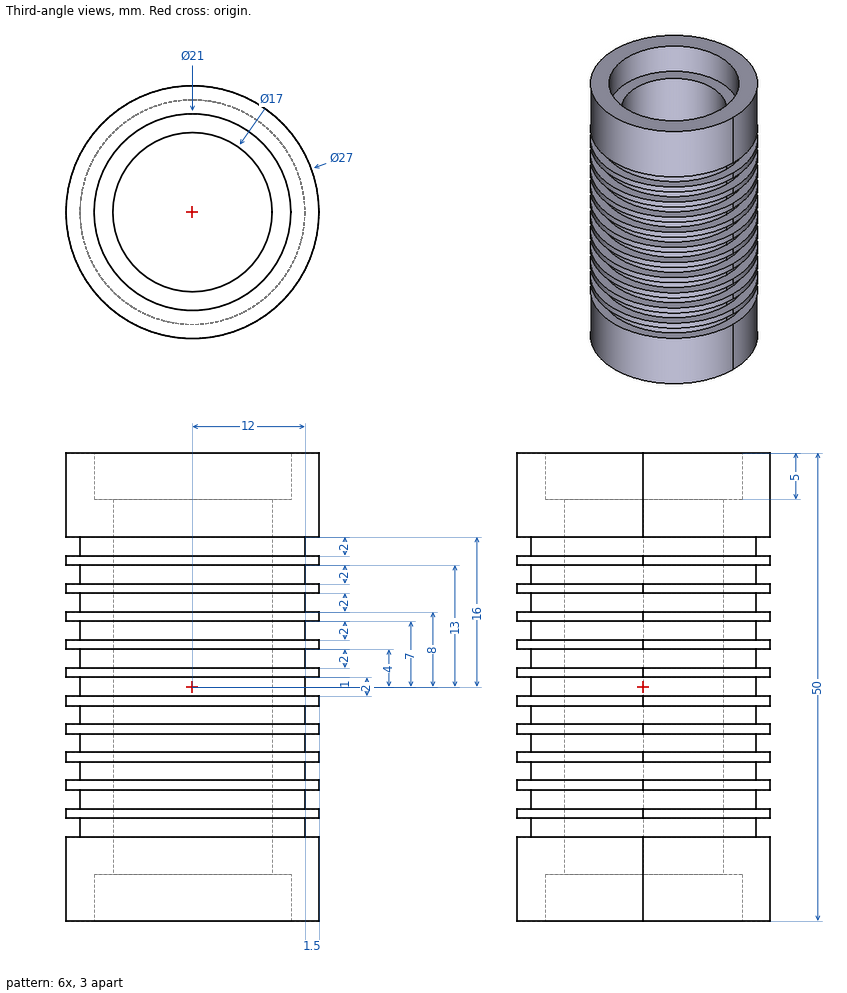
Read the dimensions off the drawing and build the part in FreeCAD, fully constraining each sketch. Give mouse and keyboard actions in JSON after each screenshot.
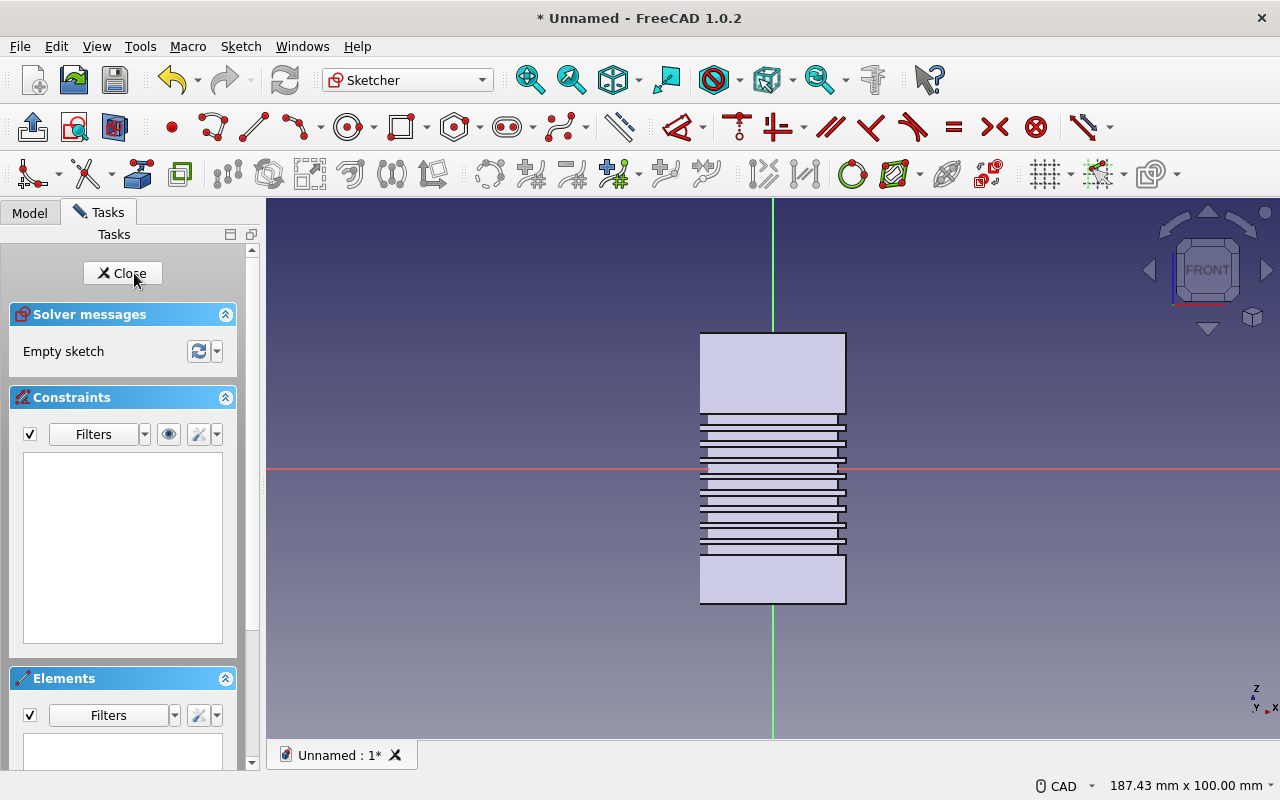
{"action": "left_click", "coordinate": [115, 128]}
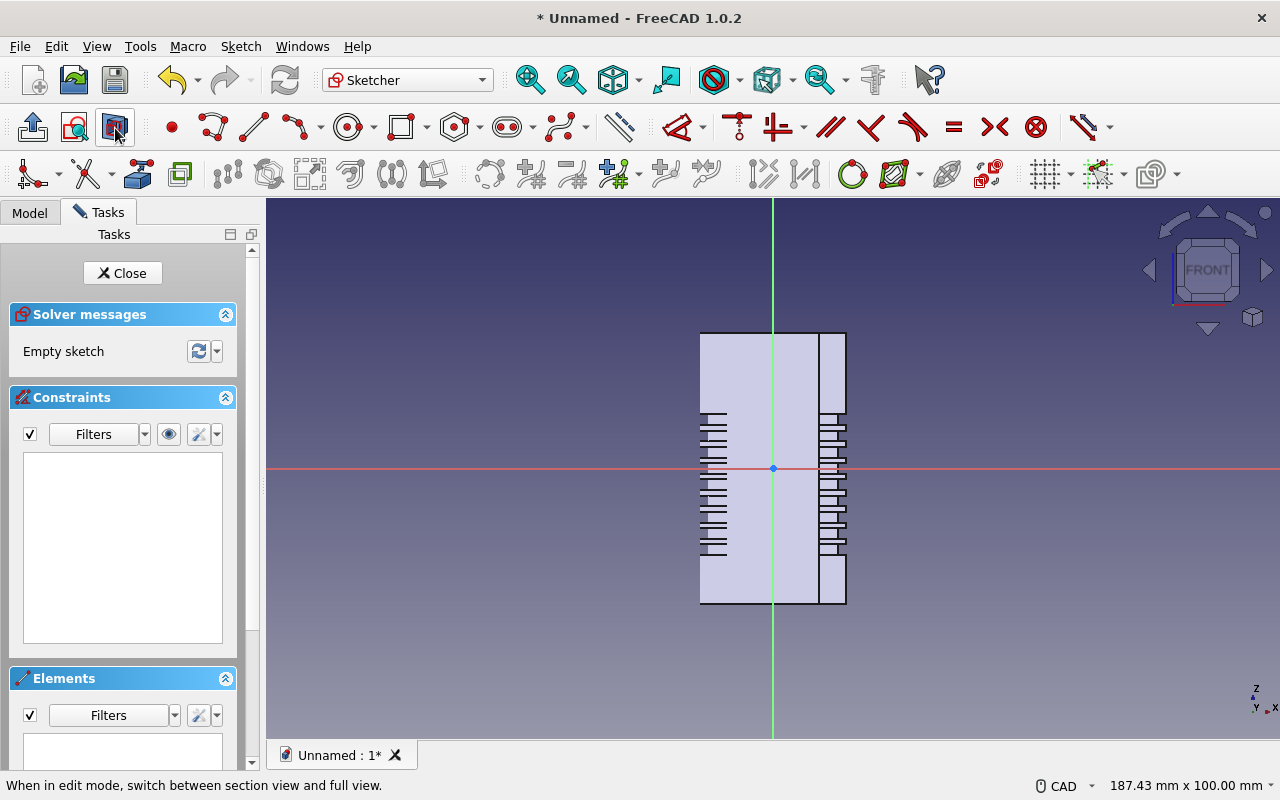
{"action": "scroll", "coordinate": [849, 400], "scroll_direction": "up", "scroll_amount": 15}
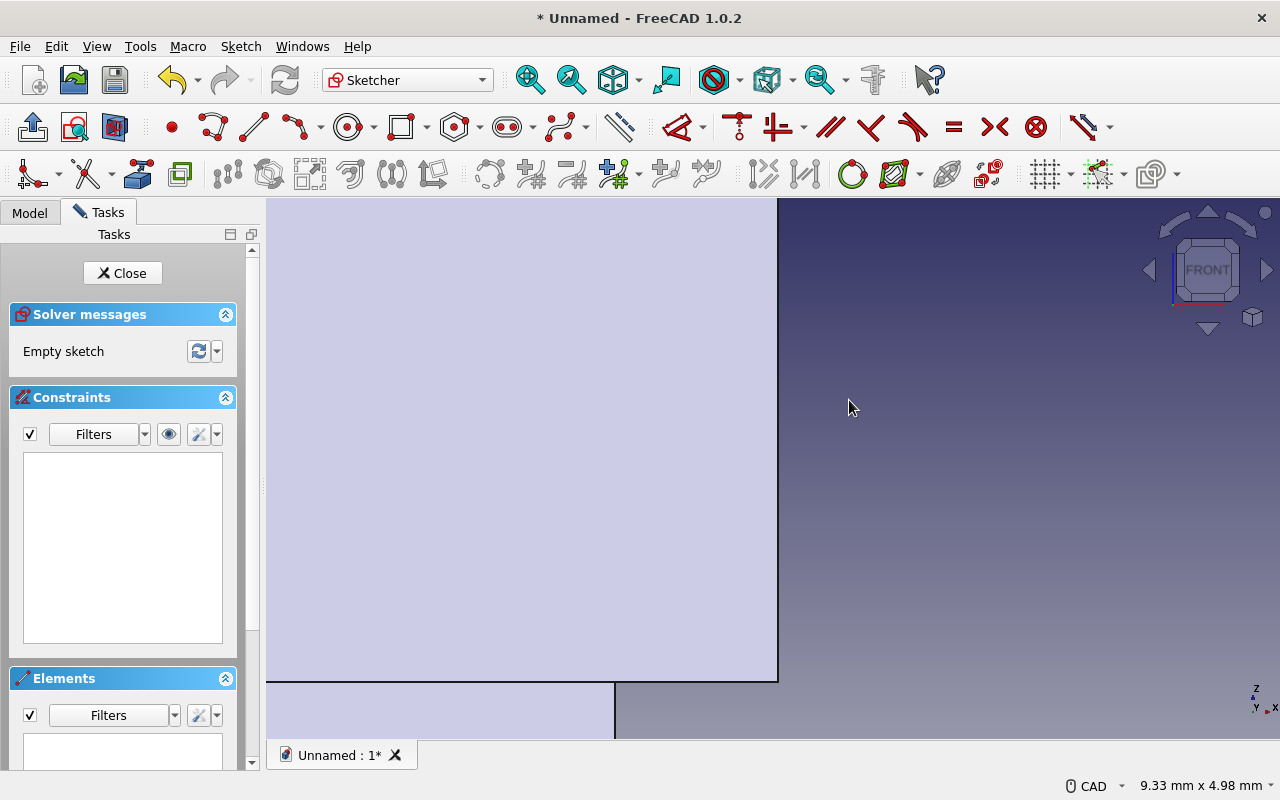
{"action": "scroll", "coordinate": [682, 457], "scroll_direction": "up", "scroll_amount": 2}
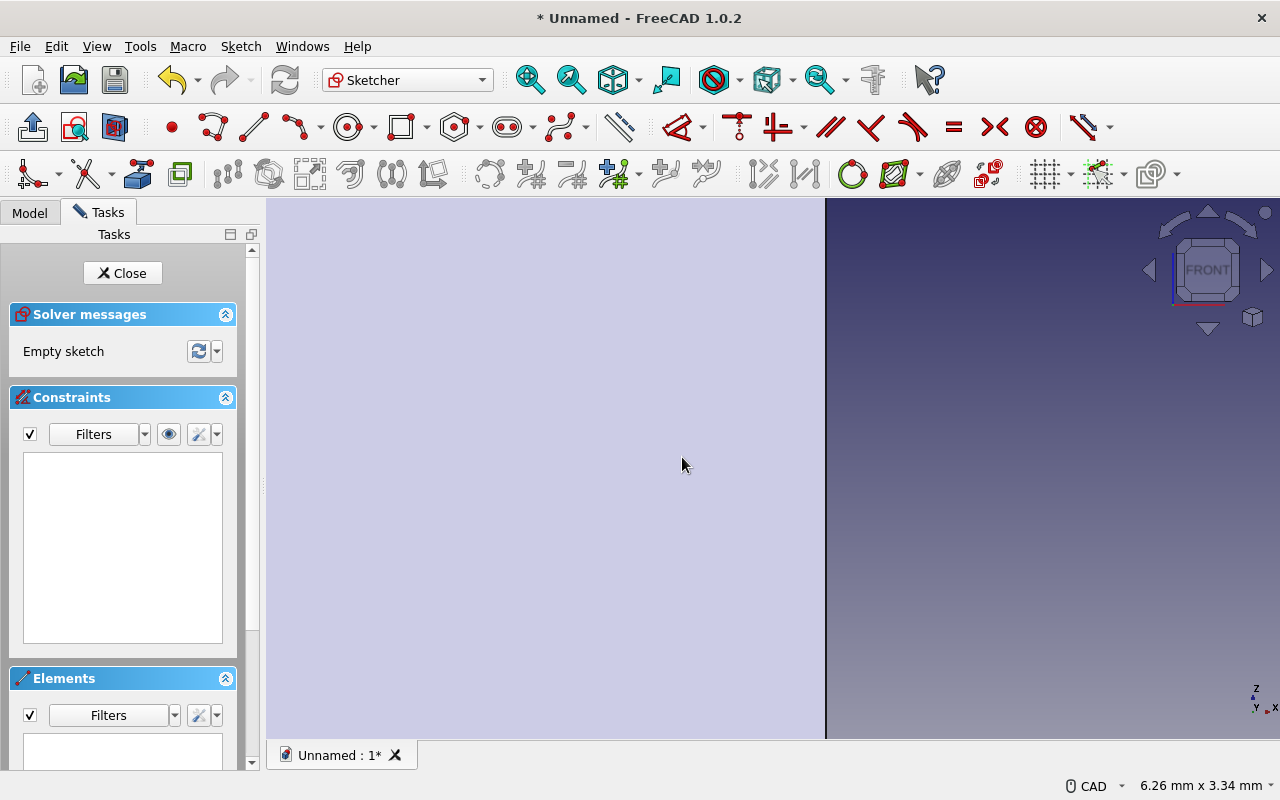
{"action": "key", "text": "g r"}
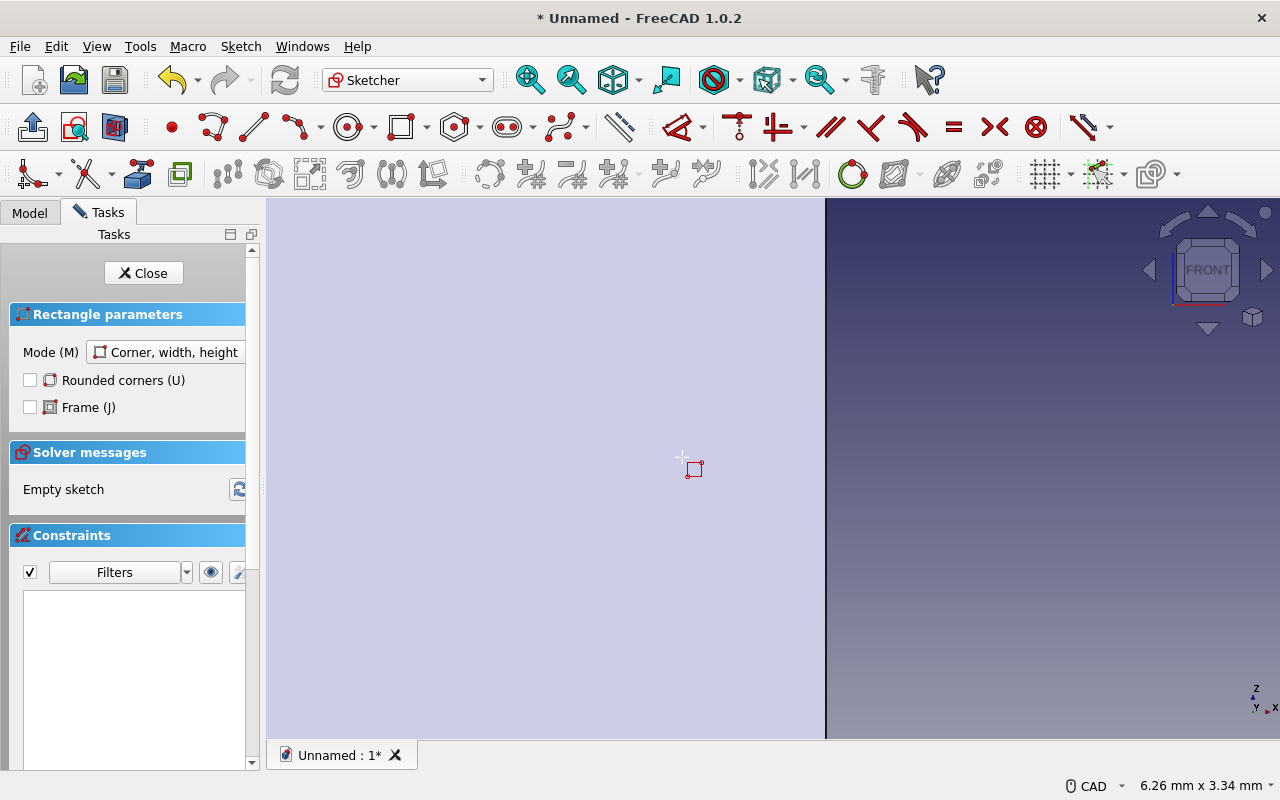
{"action": "left_click", "coordinate": [583, 306]}
{"action": "mouse_move", "coordinate": [826, 630]}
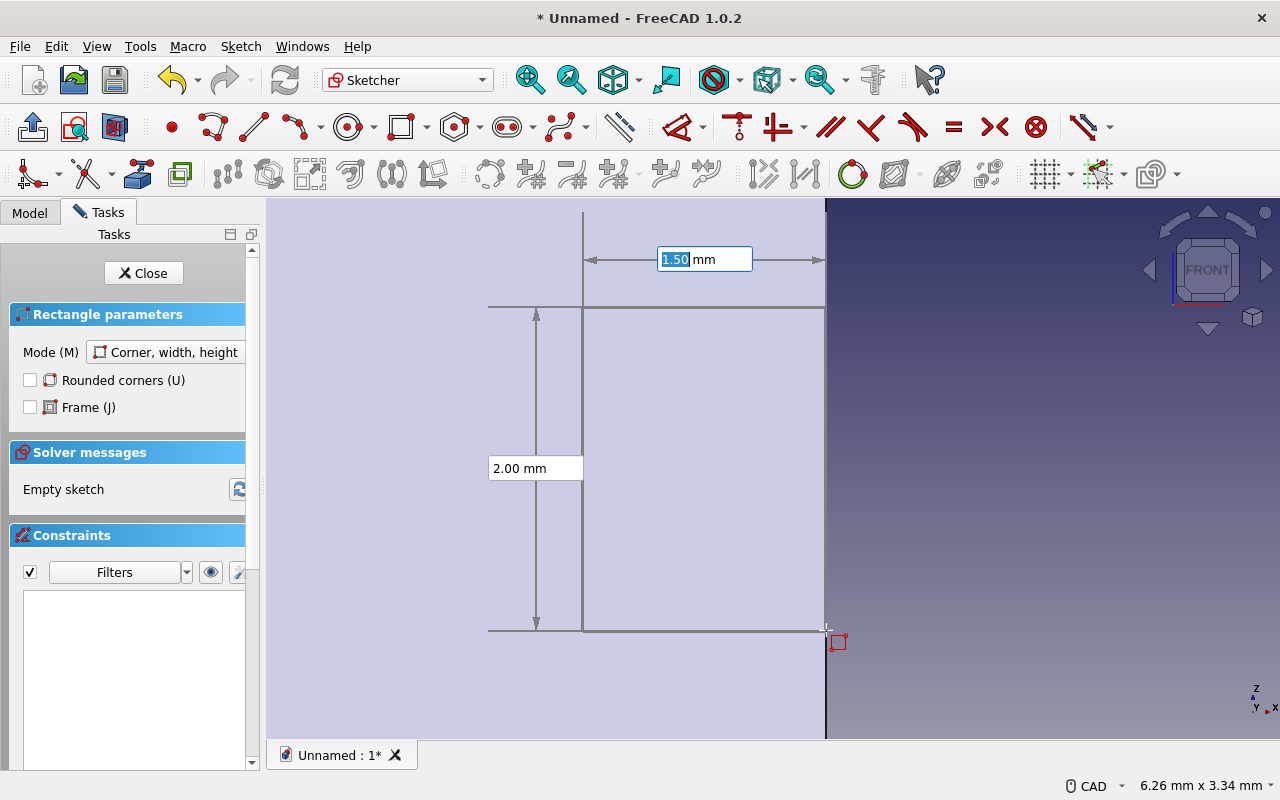
{"action": "type", "text": "1.5"}
{"action": "key", "text": "Tab"}
{"action": "type", "text": "2"}
{"action": "key", "text": "Return"}
{"action": "key", "text": "Escape"}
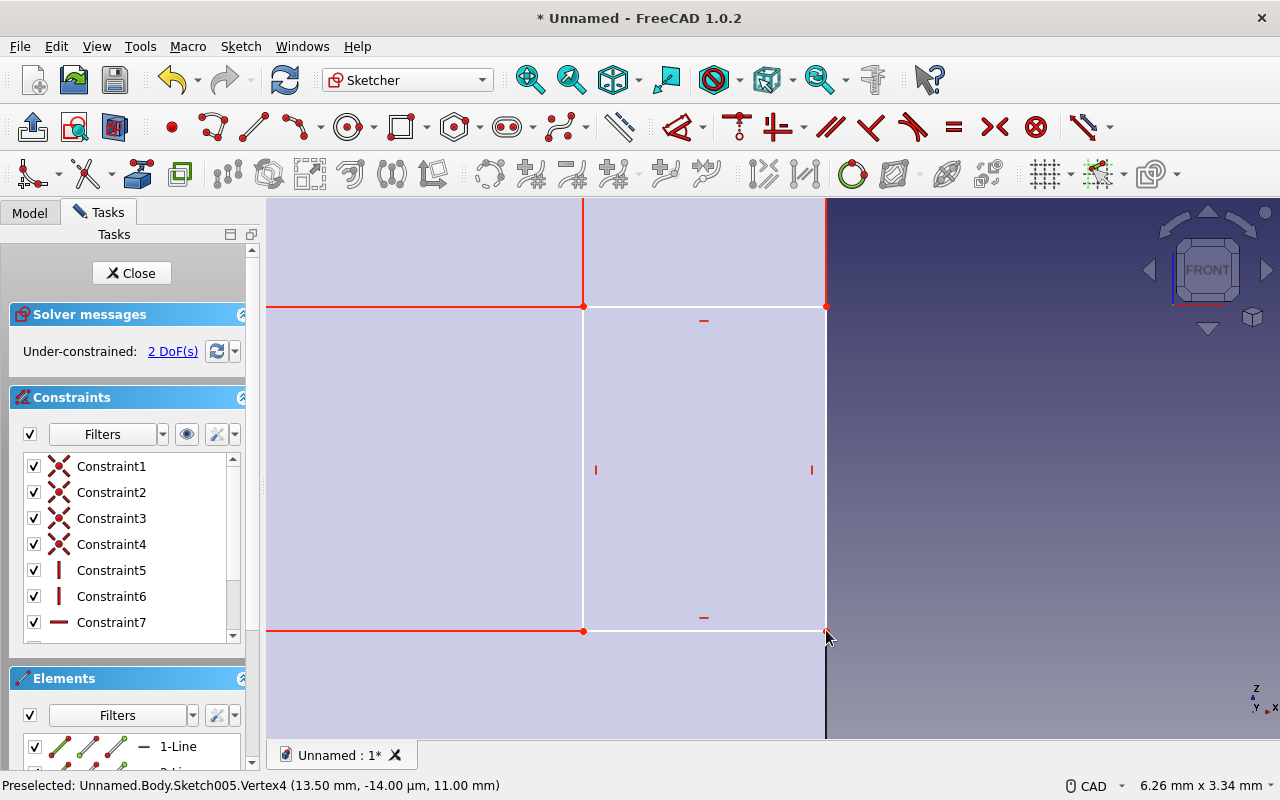
{"action": "left_click", "coordinate": [676, 128]}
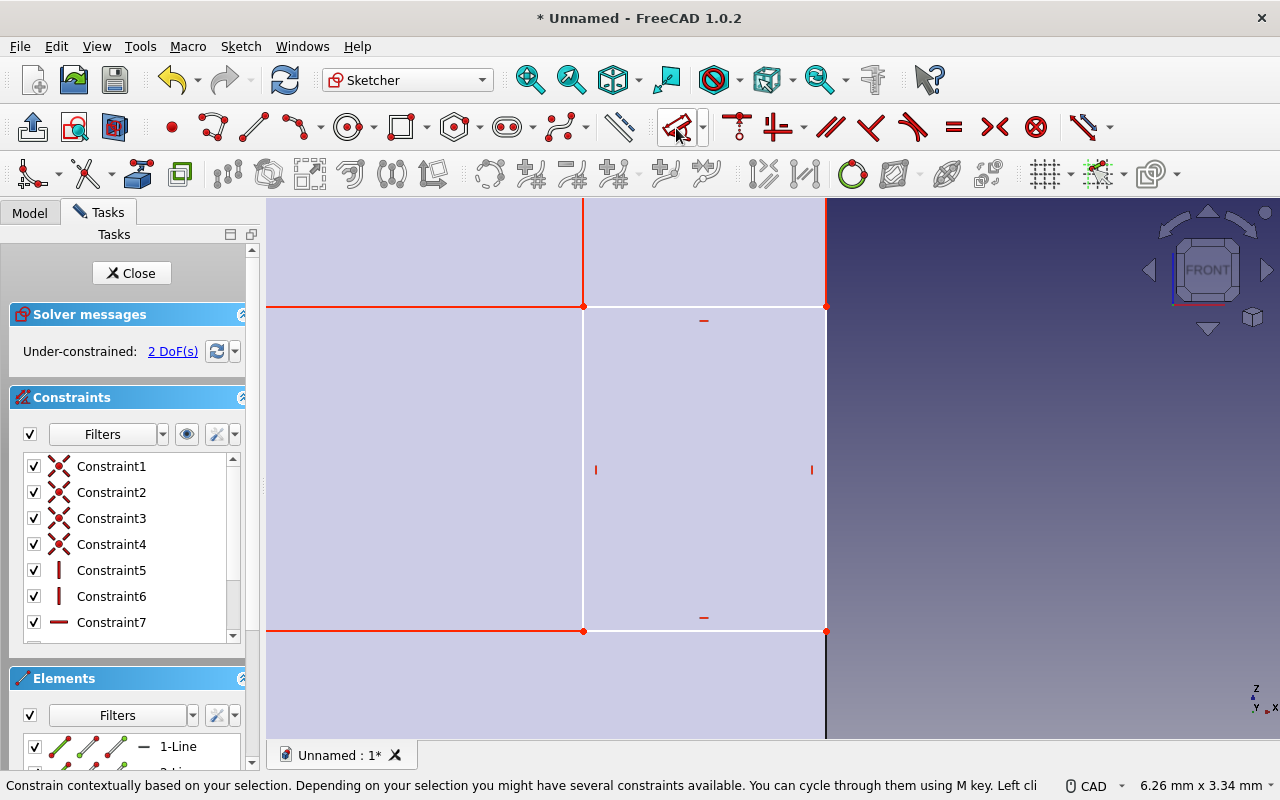
{"action": "left_click", "coordinate": [583, 307]}
{"action": "left_click", "coordinate": [438, 273]}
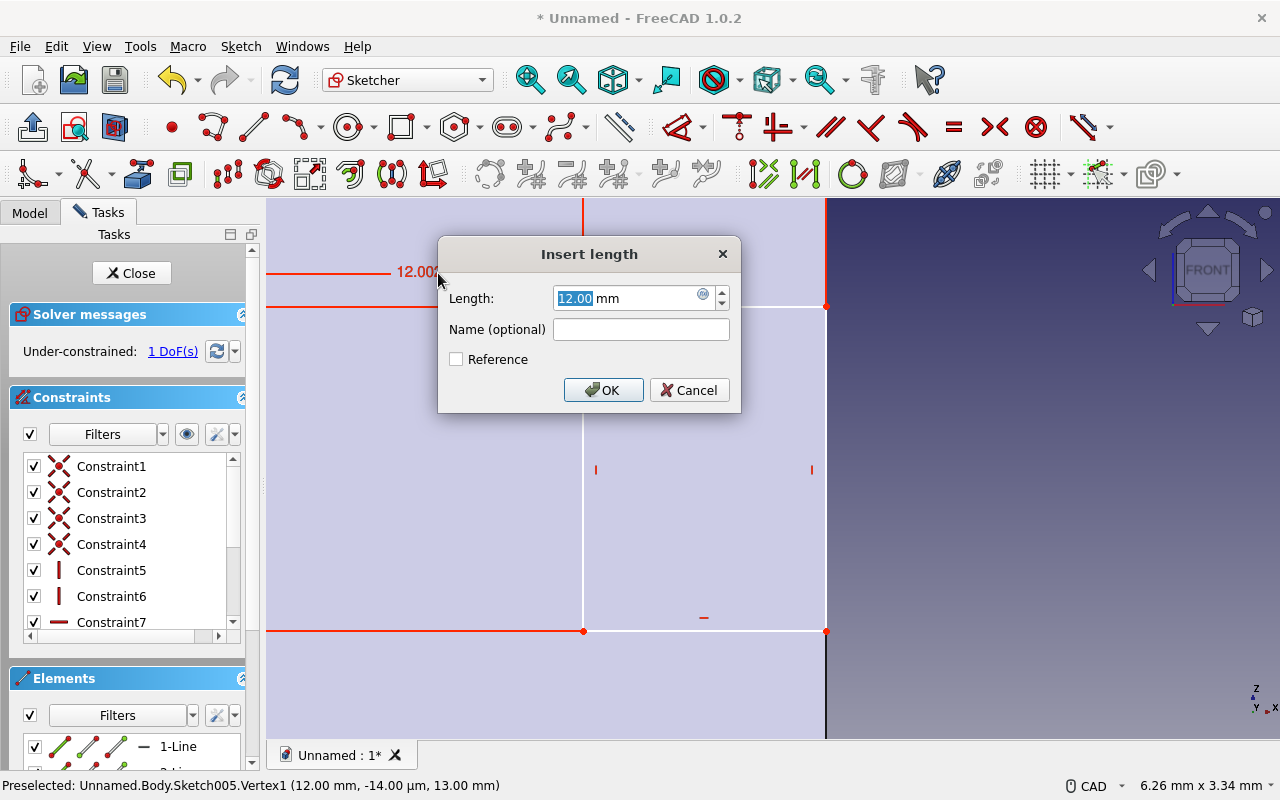
{"action": "type", "text": "12"}
{"action": "key", "text": "Return"}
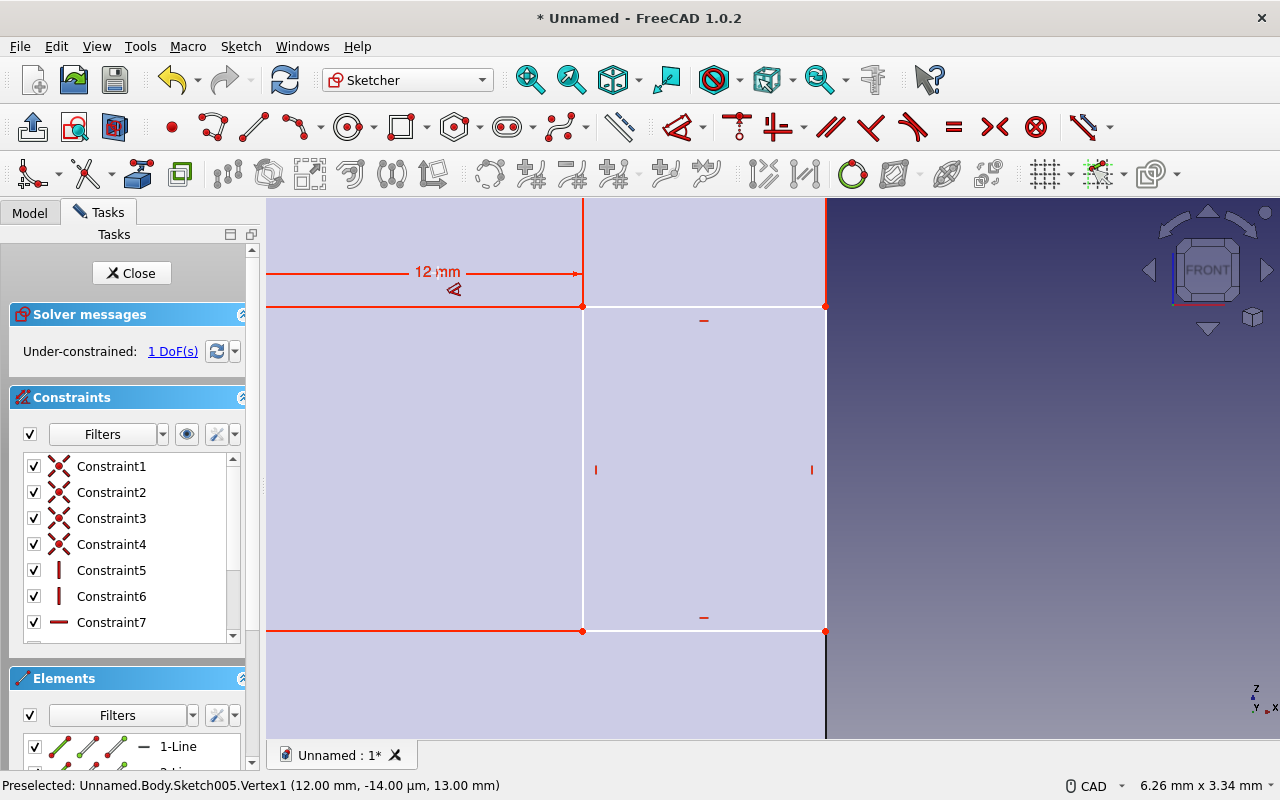
{"action": "left_click", "coordinate": [583, 307]}
{"action": "left_click", "coordinate": [617, 509]}